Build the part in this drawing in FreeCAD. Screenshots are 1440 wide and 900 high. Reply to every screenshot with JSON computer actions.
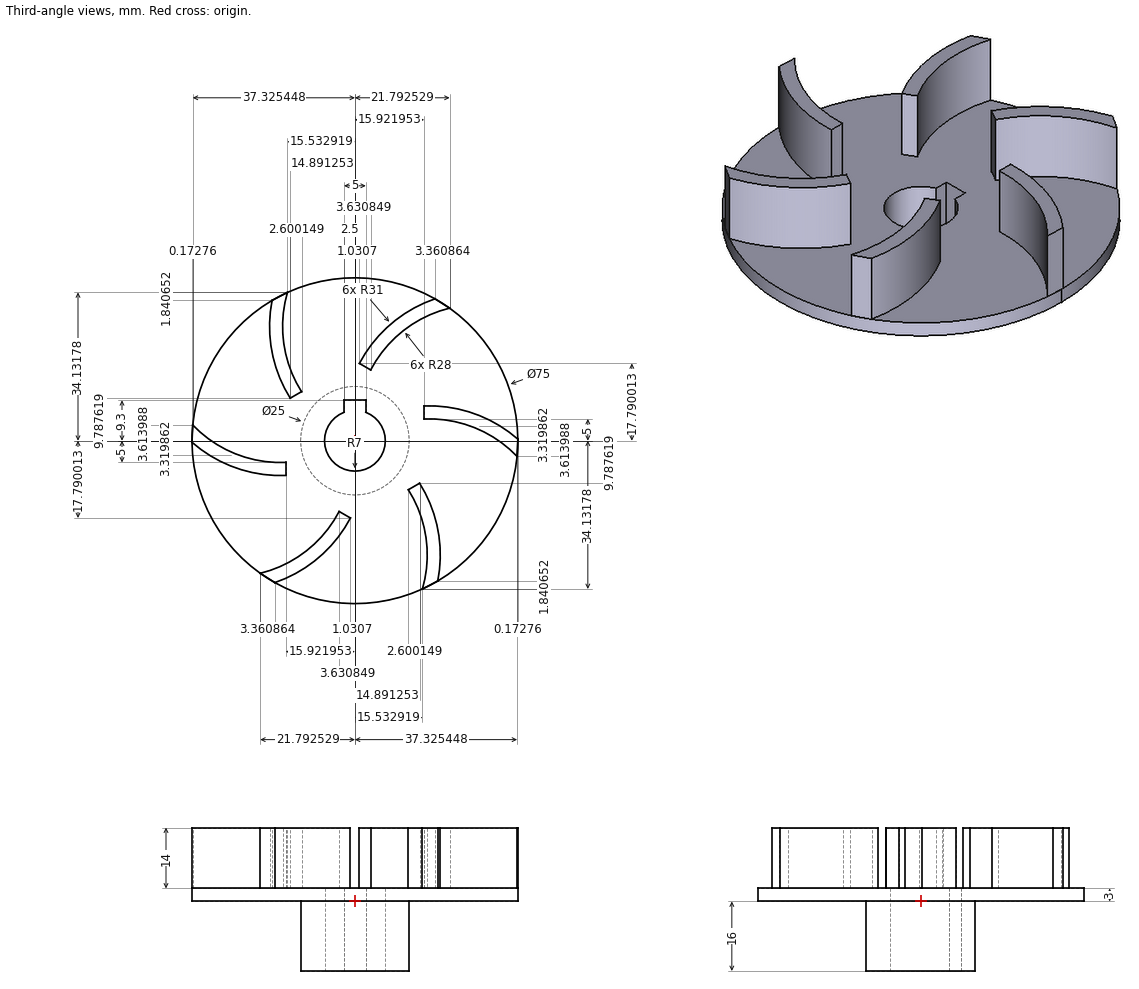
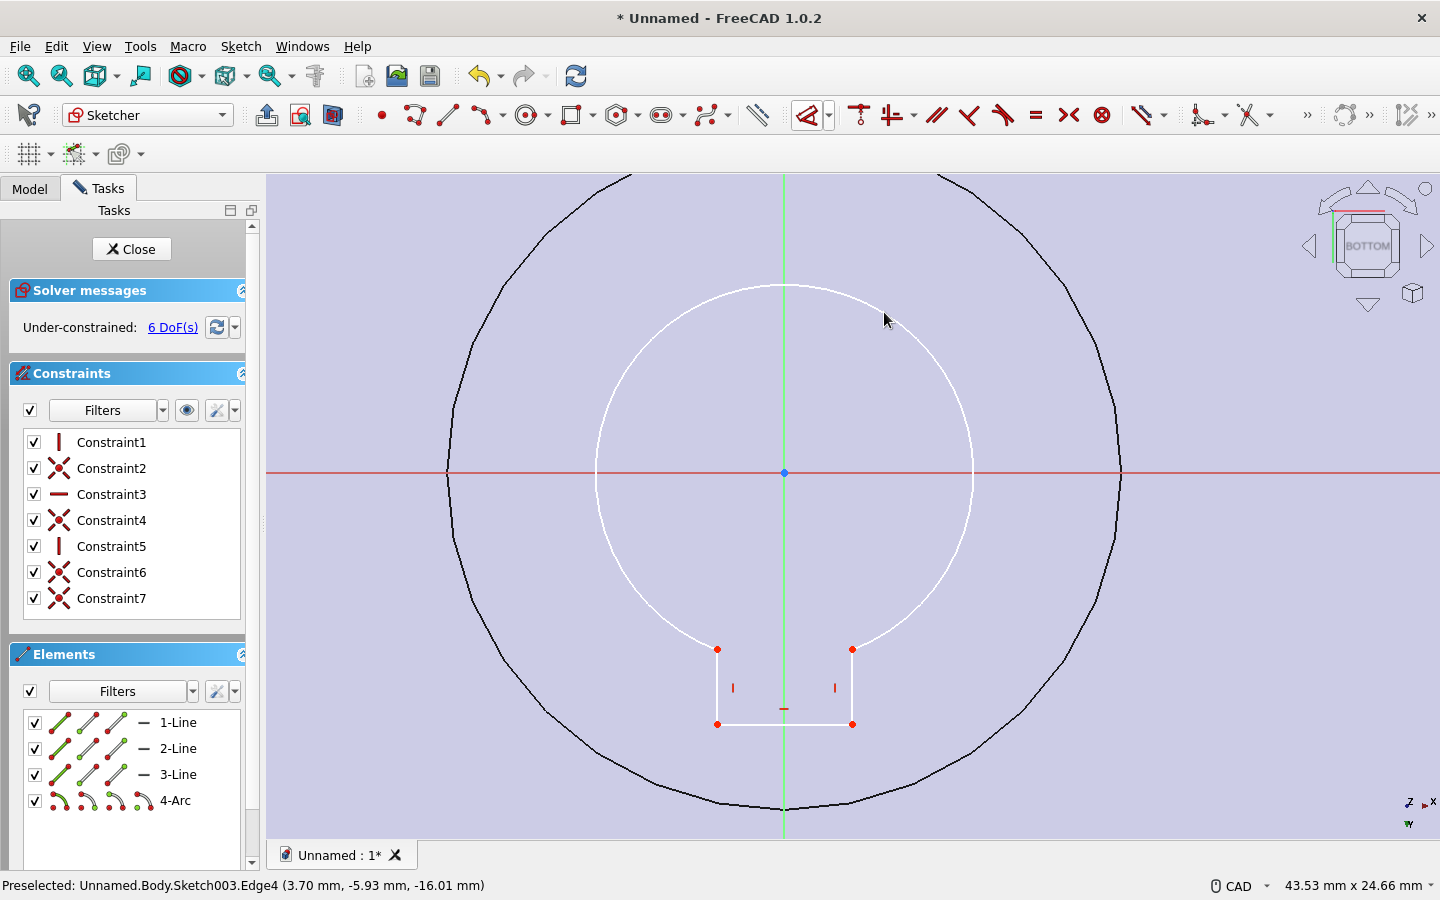
{"action": "left_click_drag", "start_coordinate": [774, 463], "coordinate": [794, 484]}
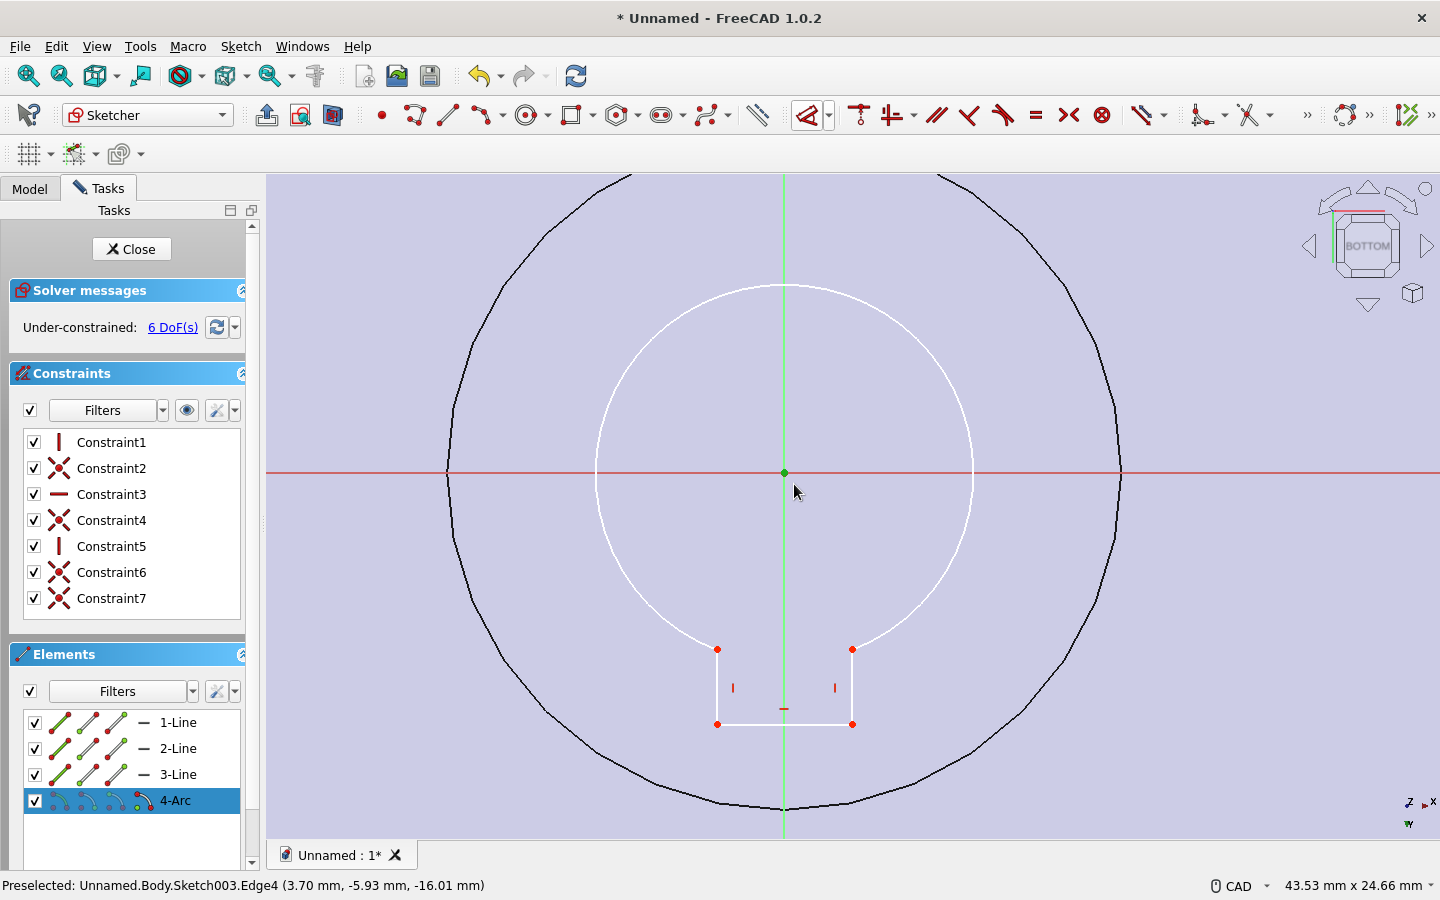
{"action": "key", "text": "c"}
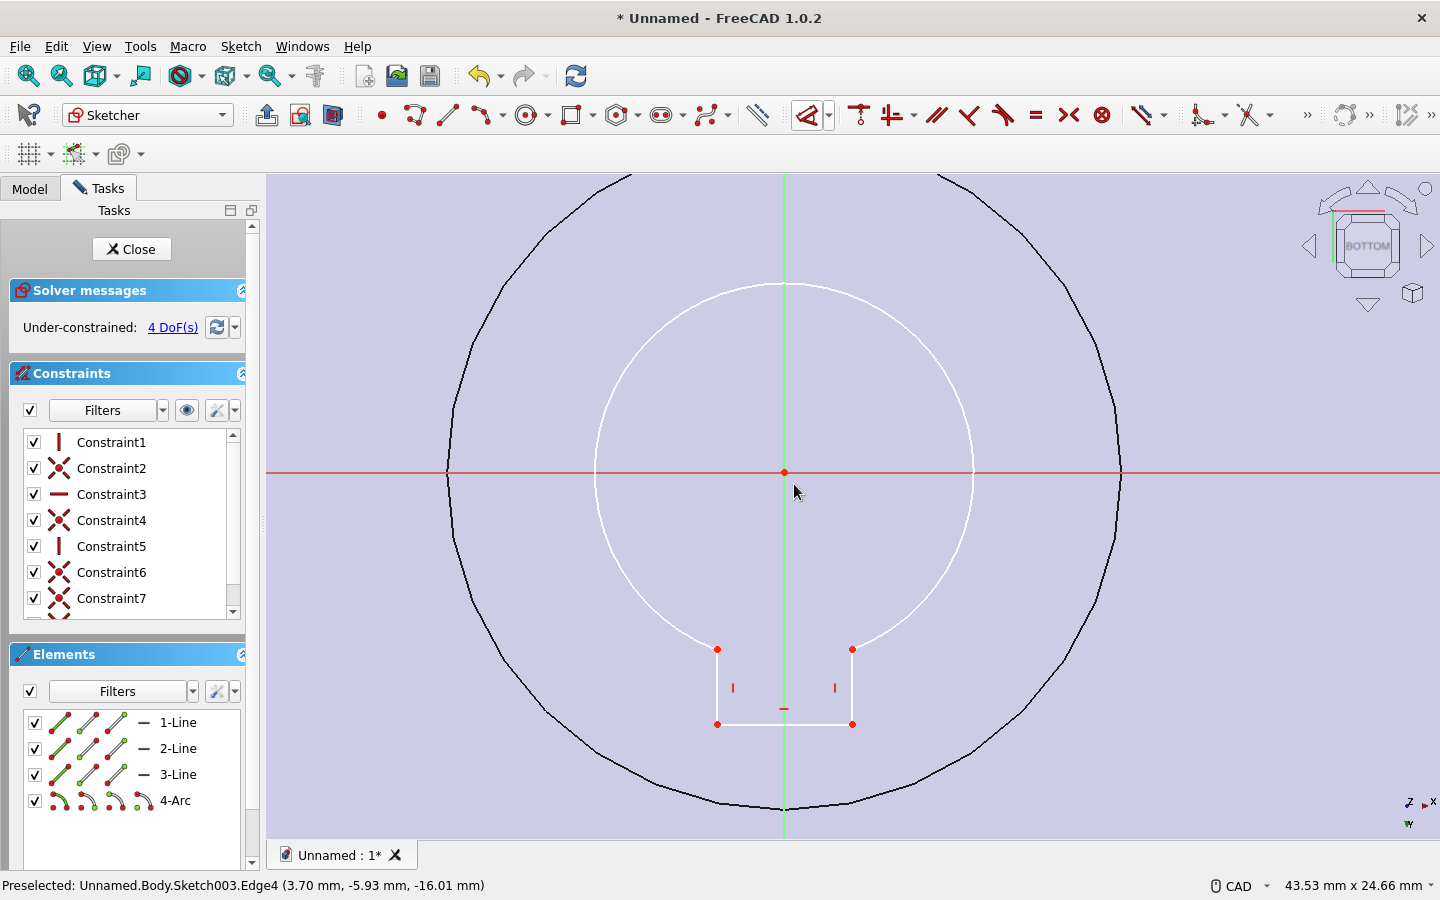
{"action": "left_click", "coordinate": [954, 388]}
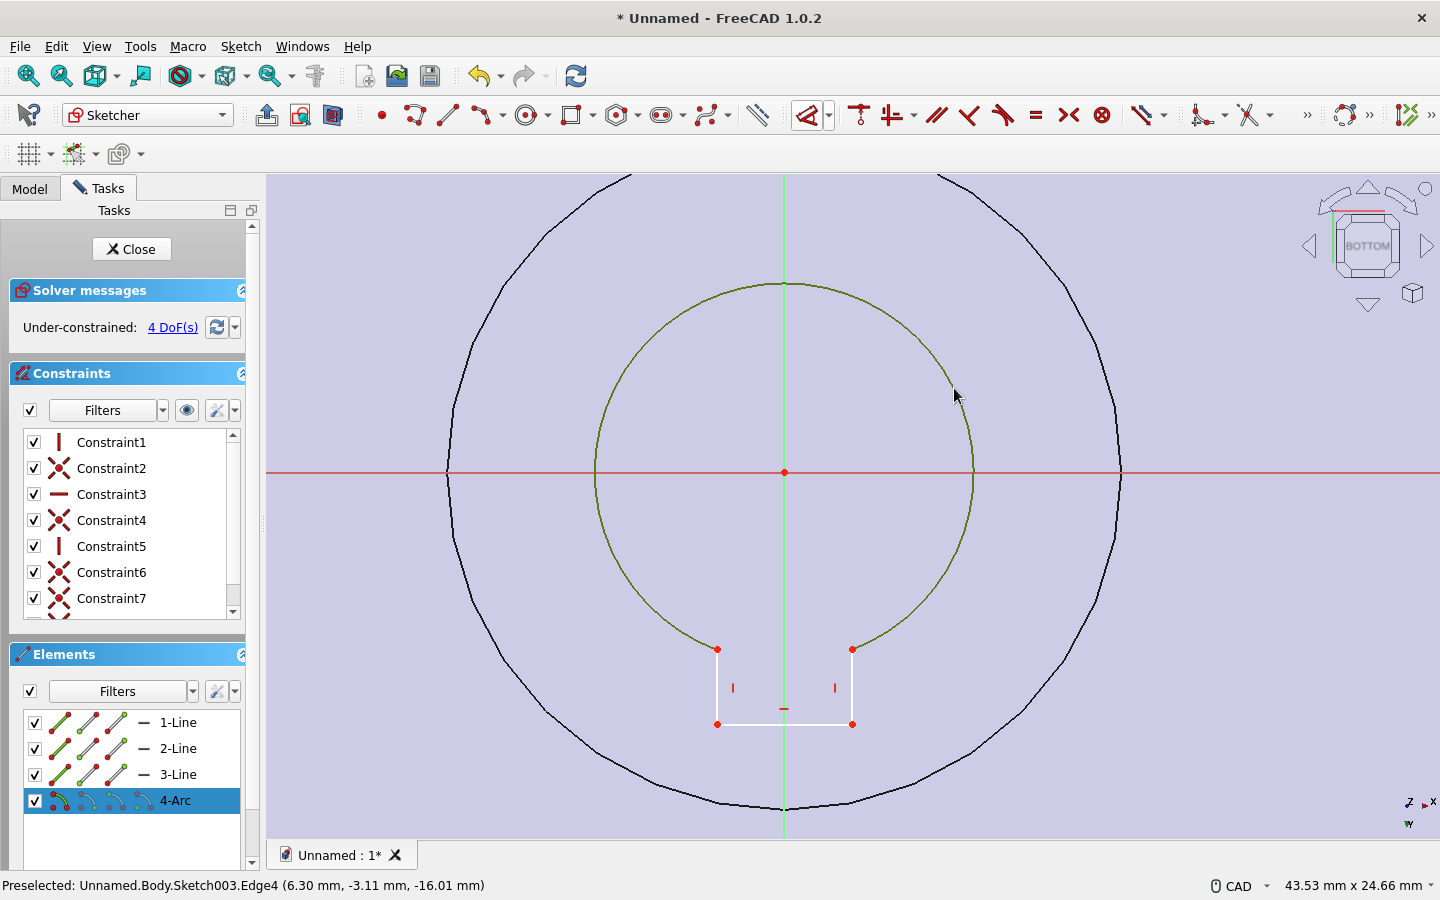
{"action": "key", "text": "k r"}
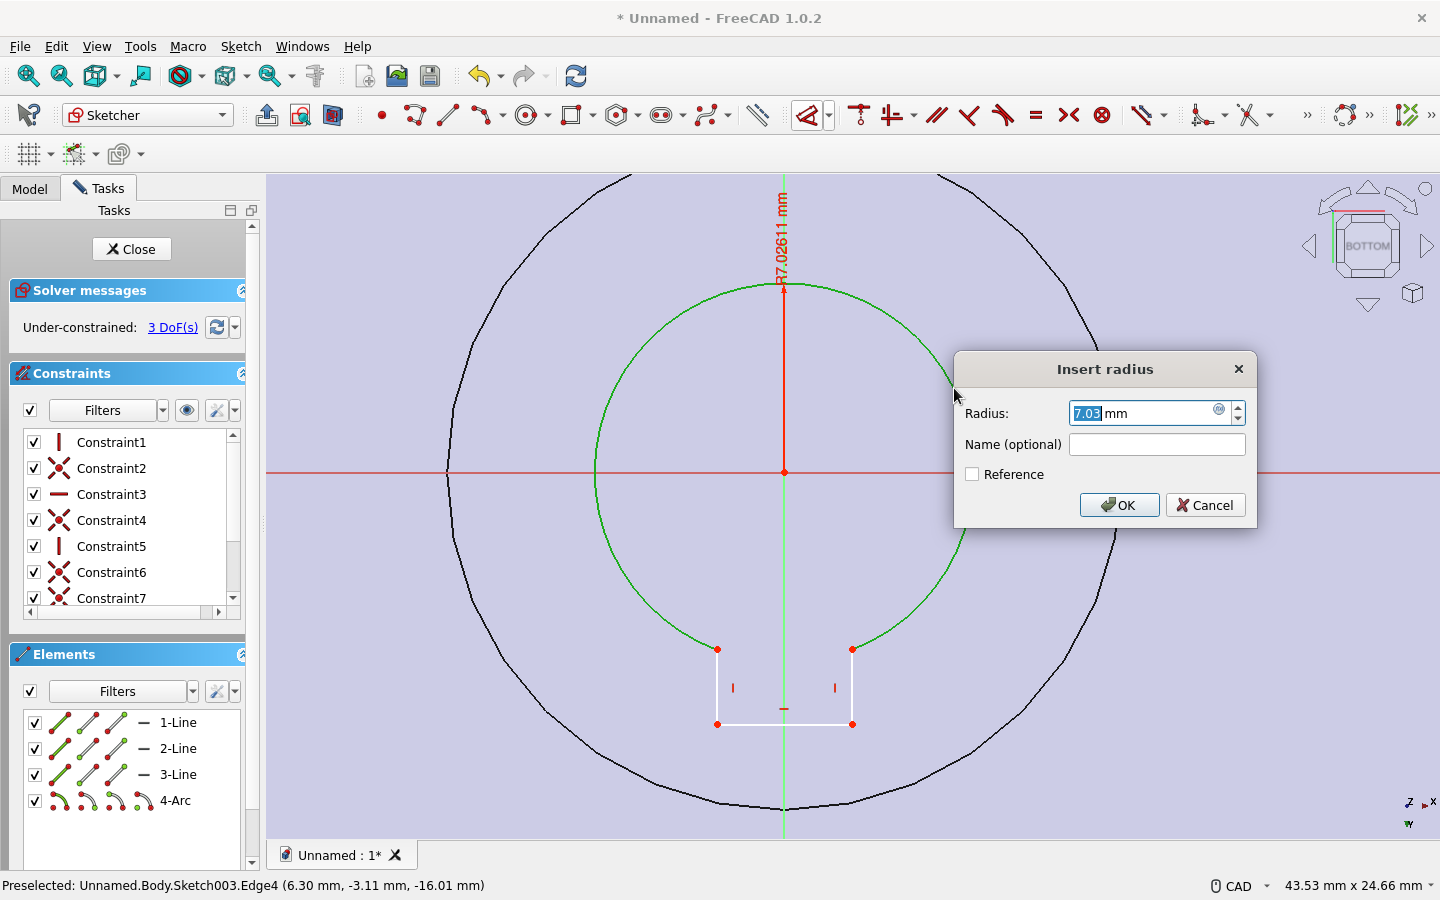
{"action": "type", "text": "7"}
{"action": "key", "text": "Return"}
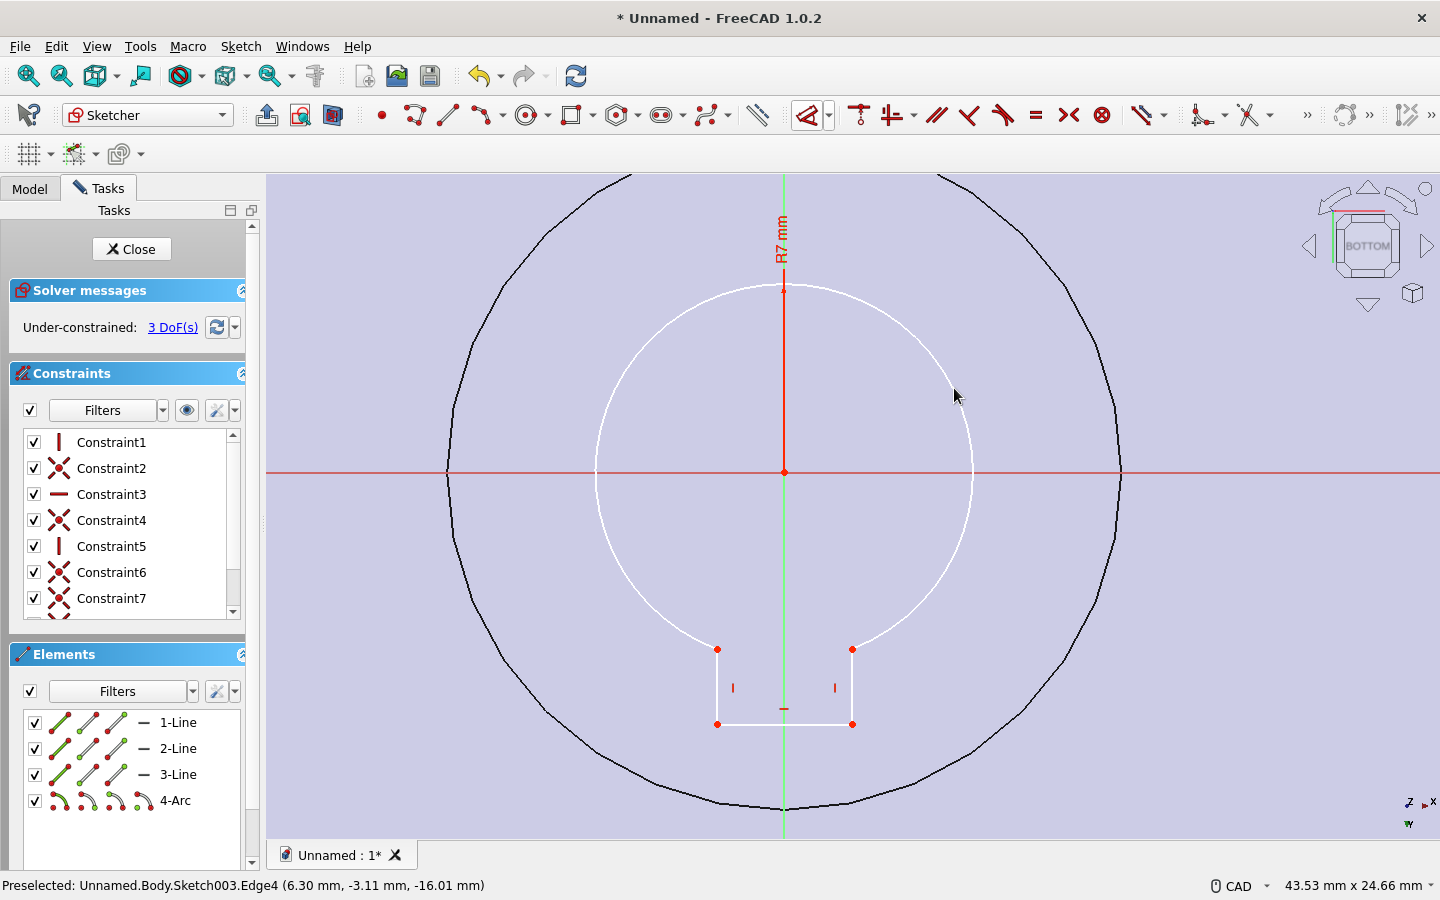
{"action": "left_click", "coordinate": [757, 725]}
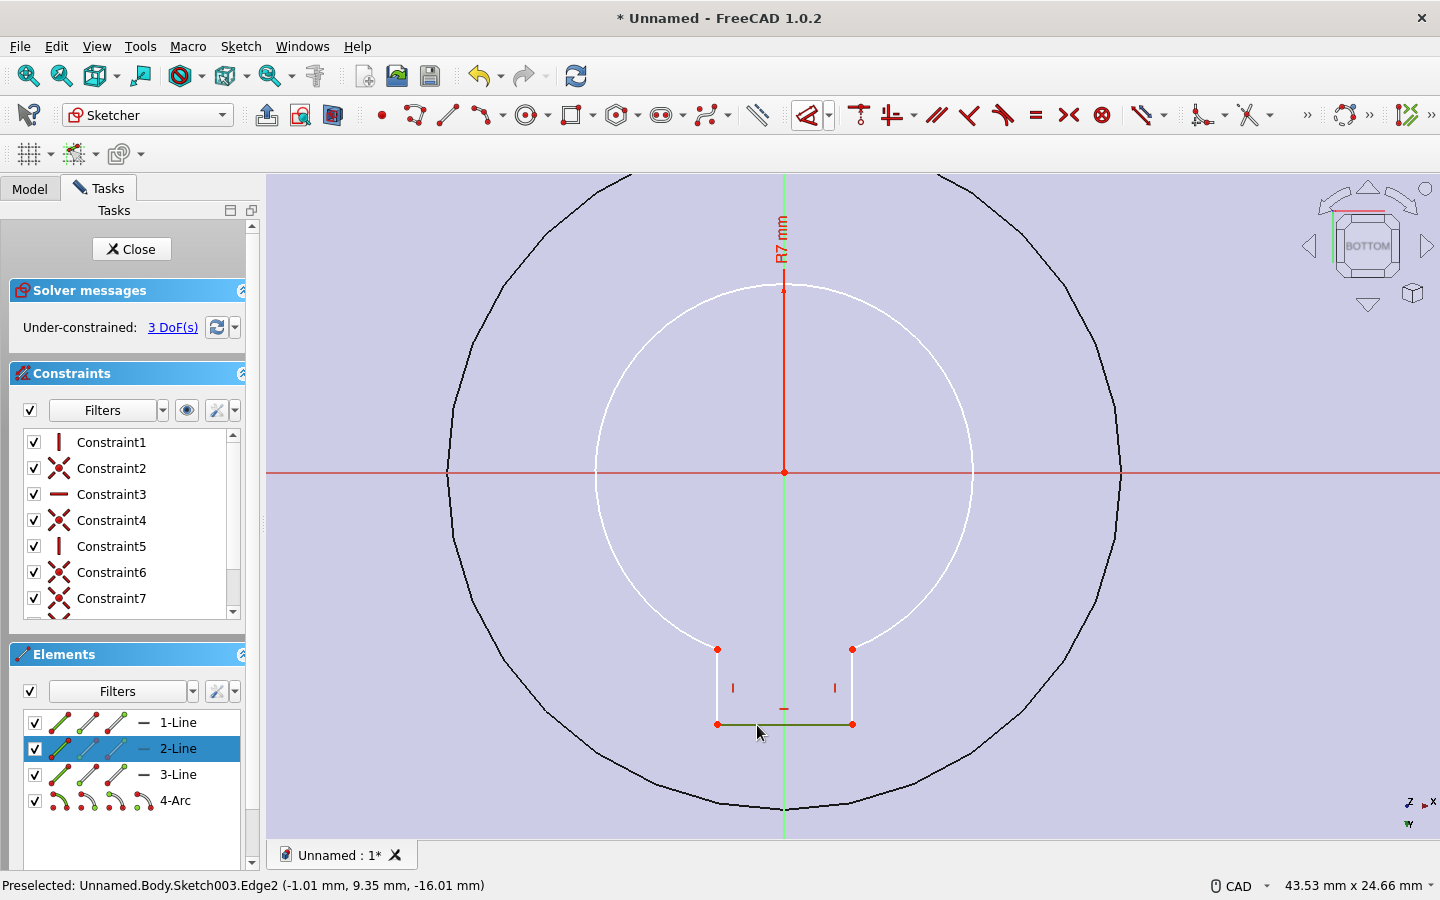
{"action": "key", "text": "l"}